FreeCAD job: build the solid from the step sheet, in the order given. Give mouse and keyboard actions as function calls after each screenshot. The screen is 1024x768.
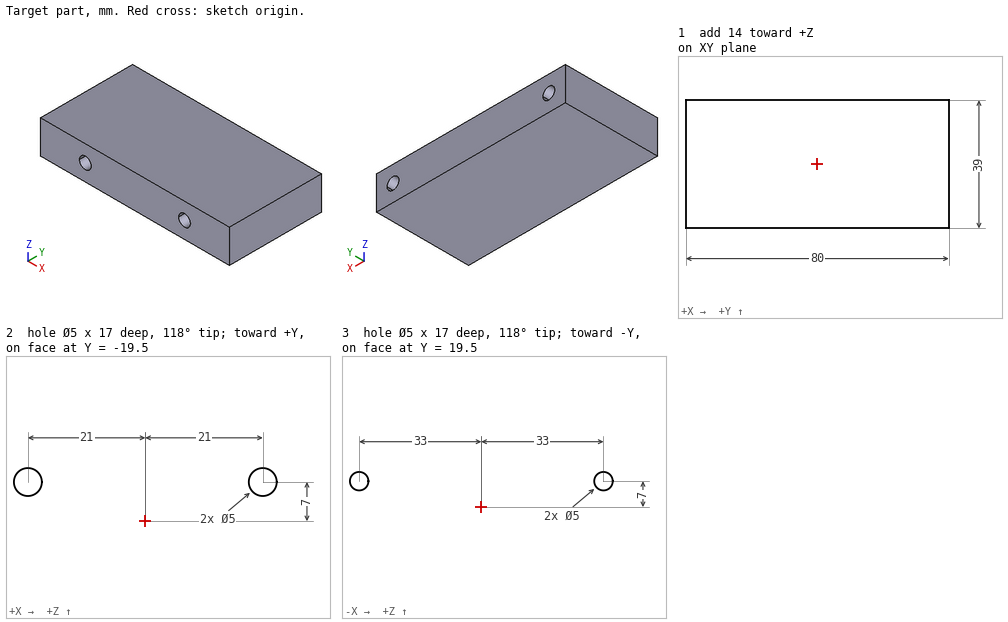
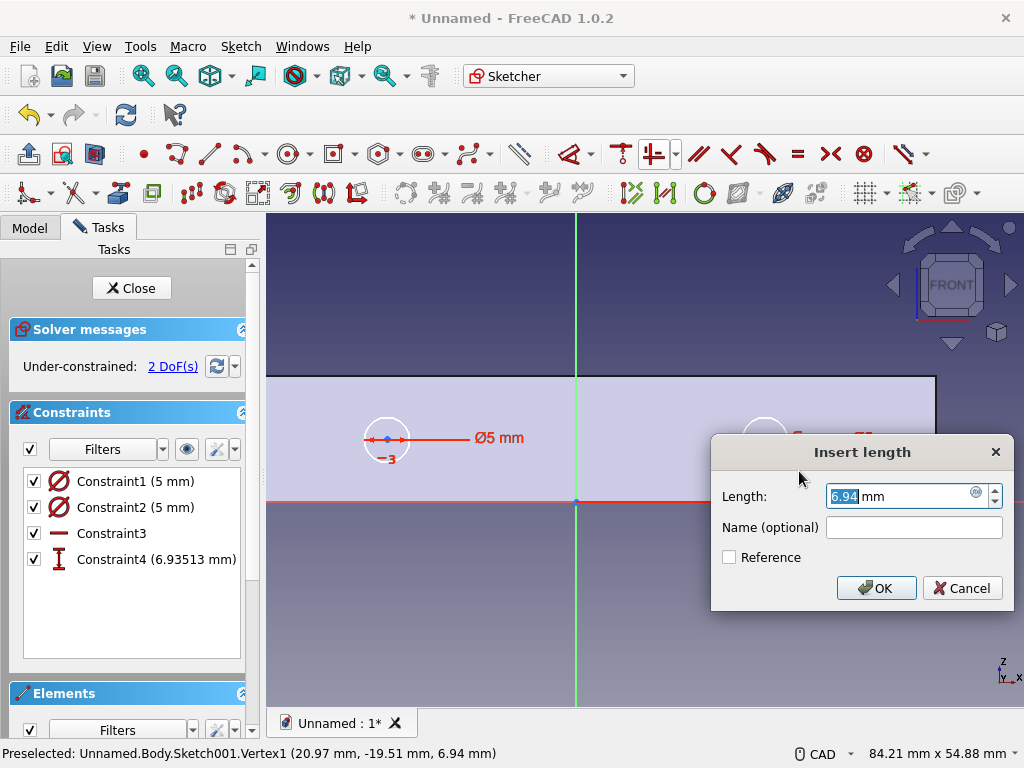
text(7)
key(Return)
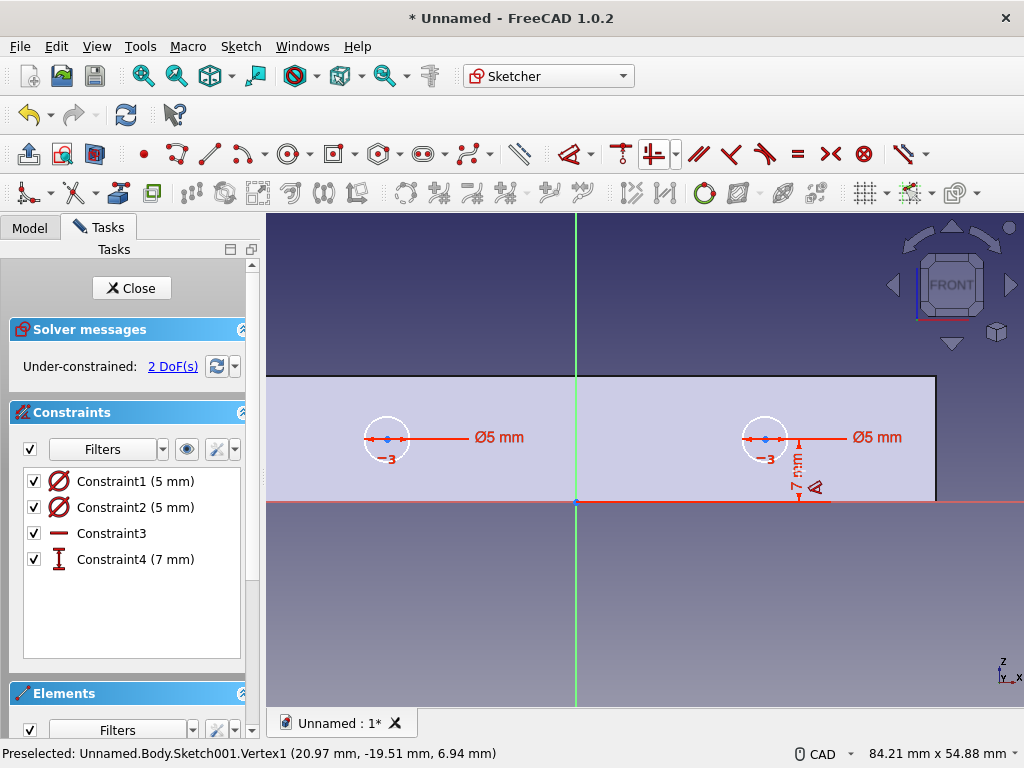
click(765, 439)
click(671, 536)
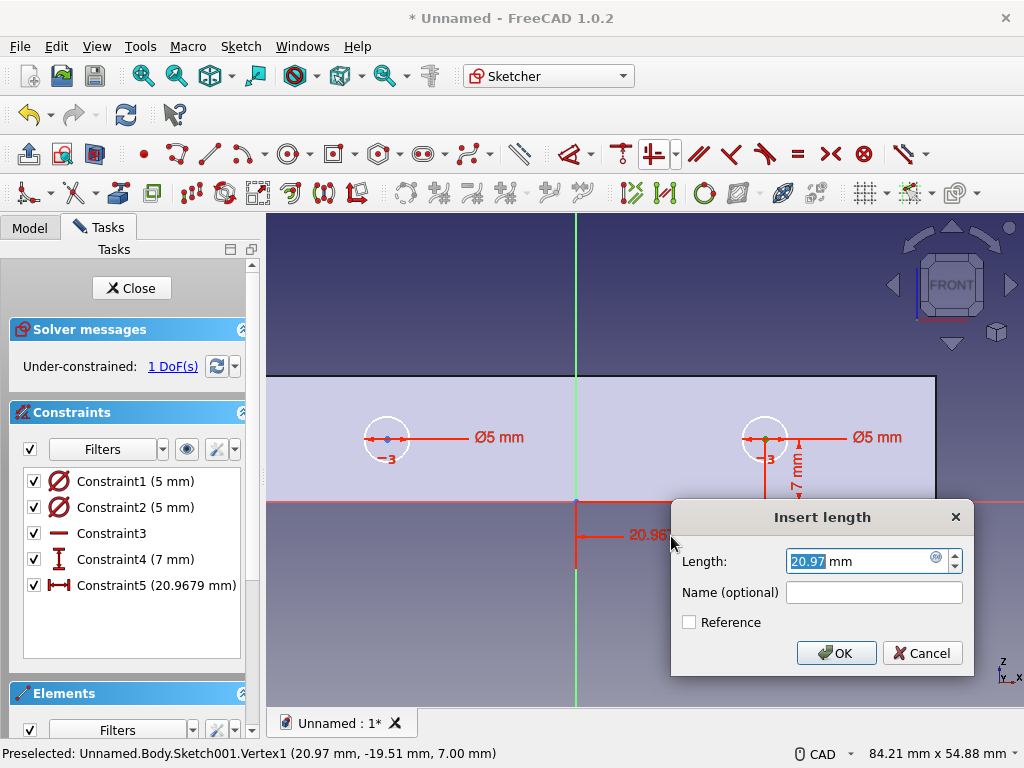
text(21)
key(Return)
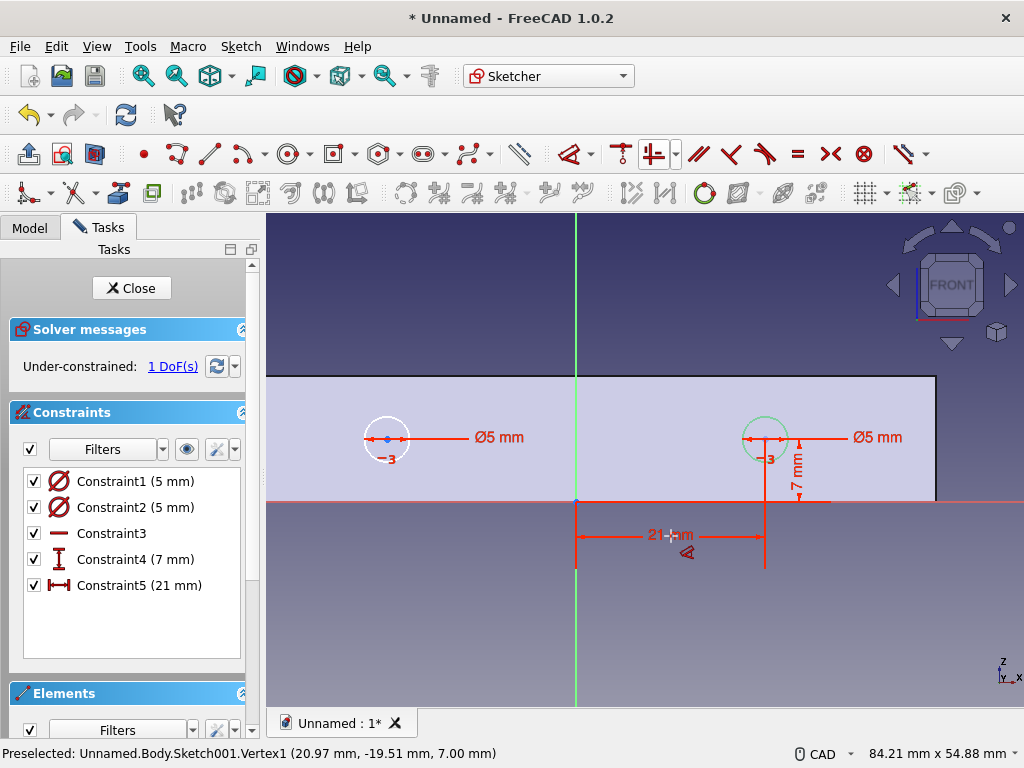
click(387, 439)
click(482, 536)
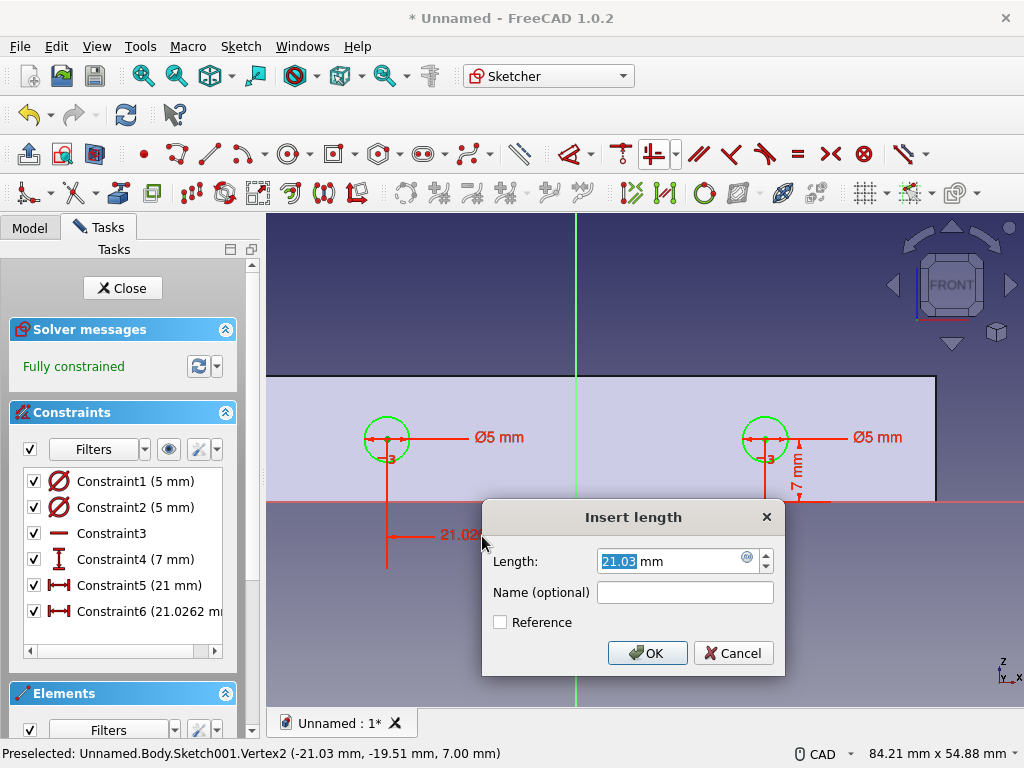
text(21)
key(Return)
key(Escape)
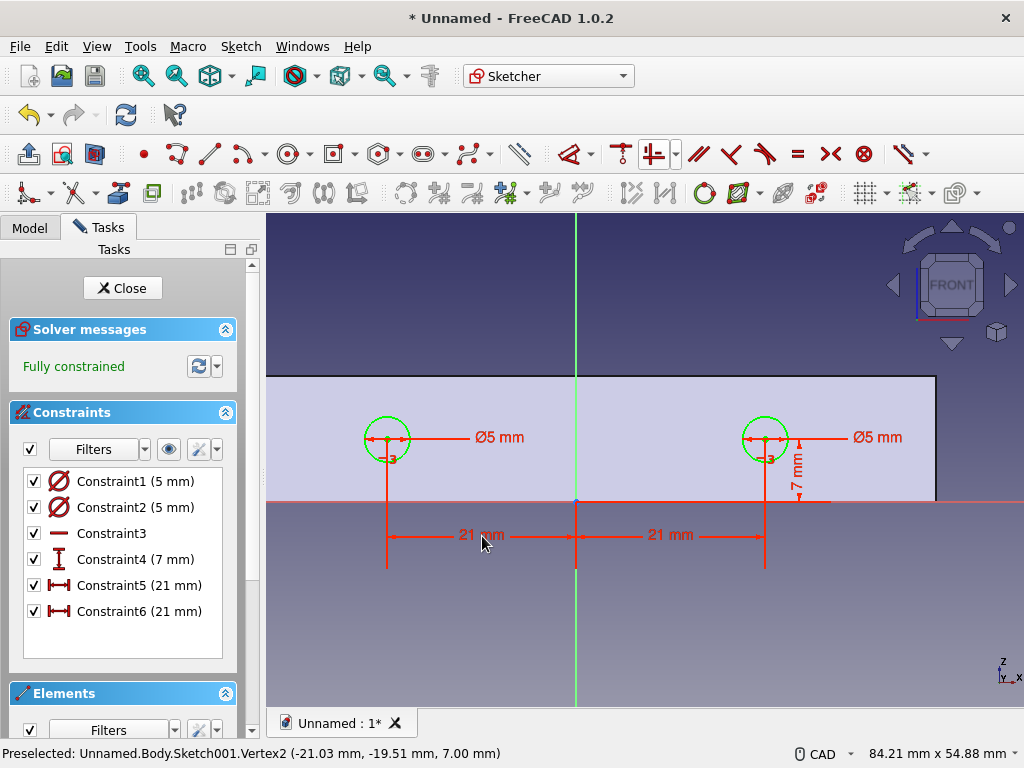
click(123, 288)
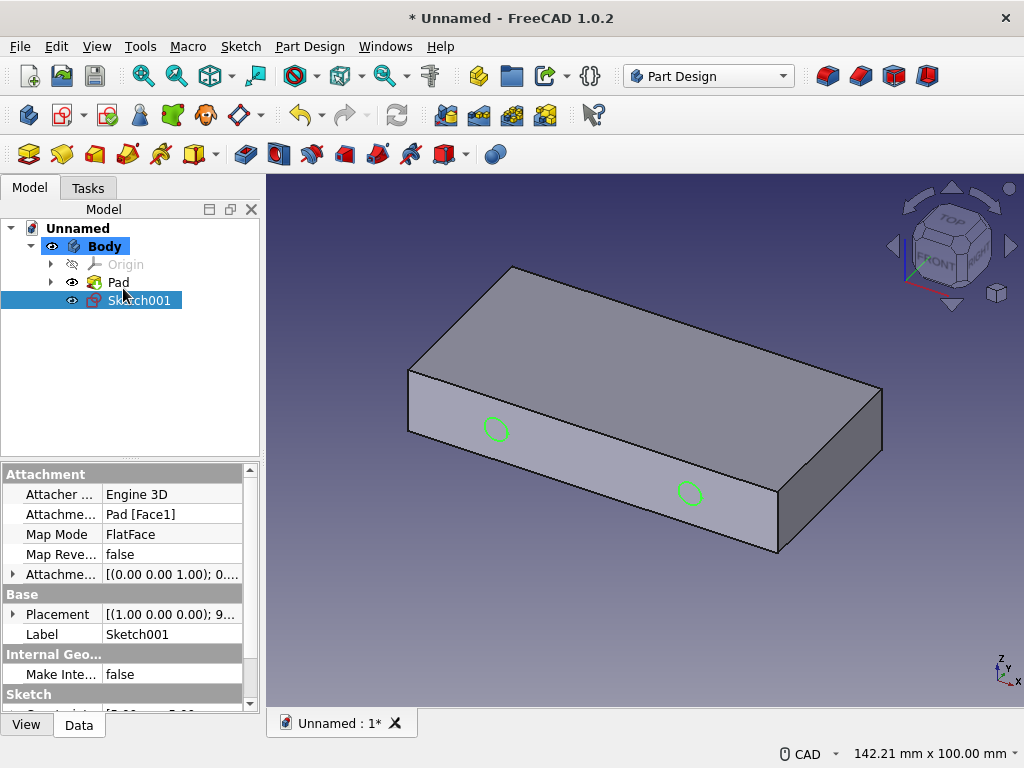
click(279, 154)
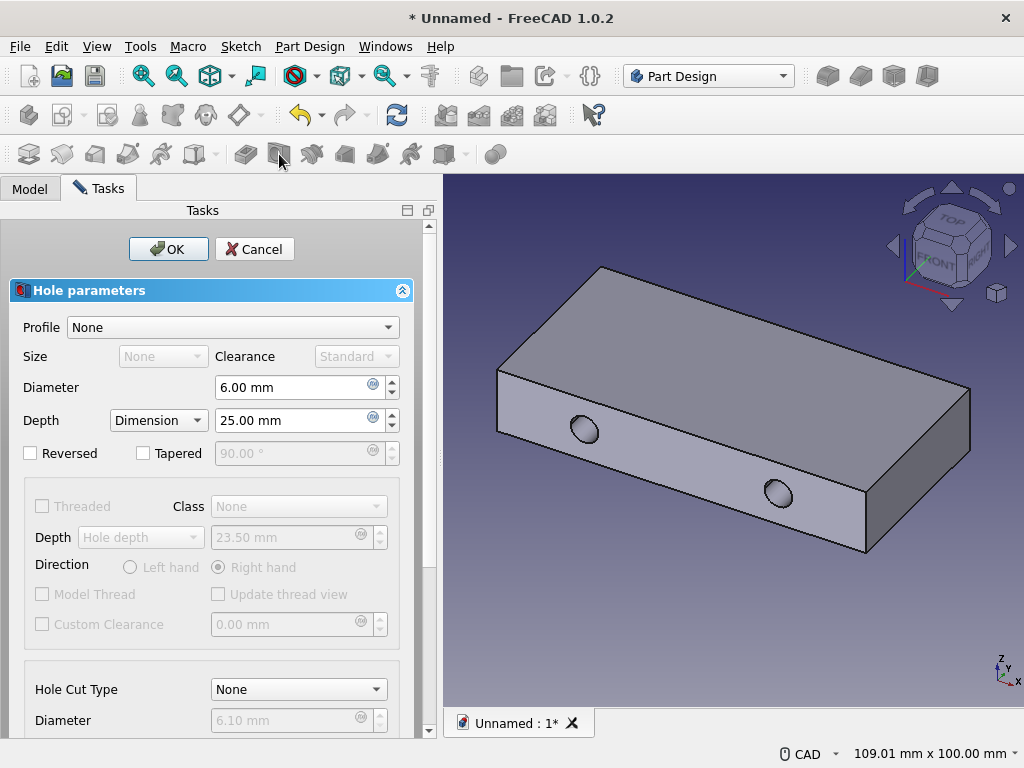
triple_click(300, 388)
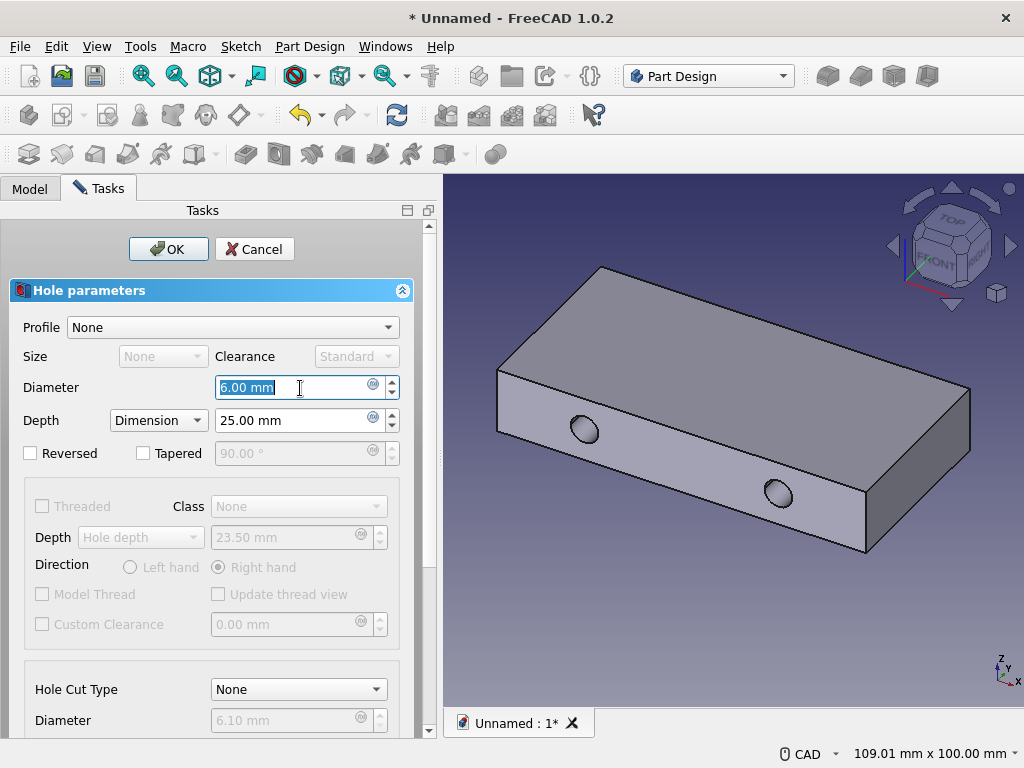
text(5)
key(Tab)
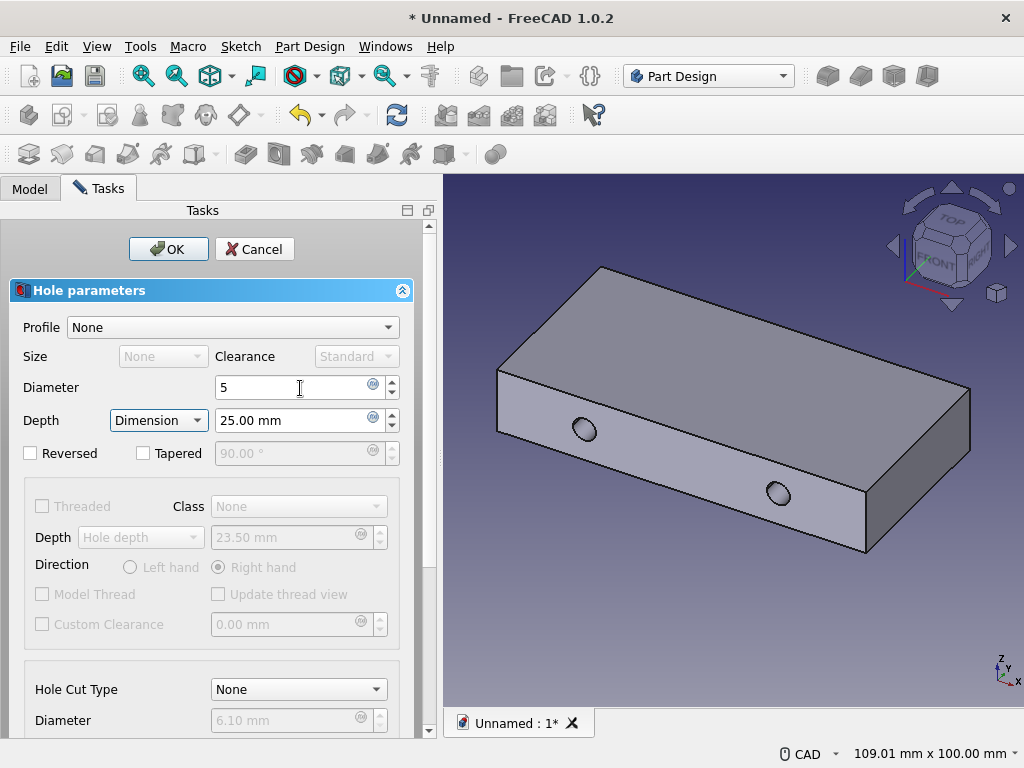
triple_click(300, 420)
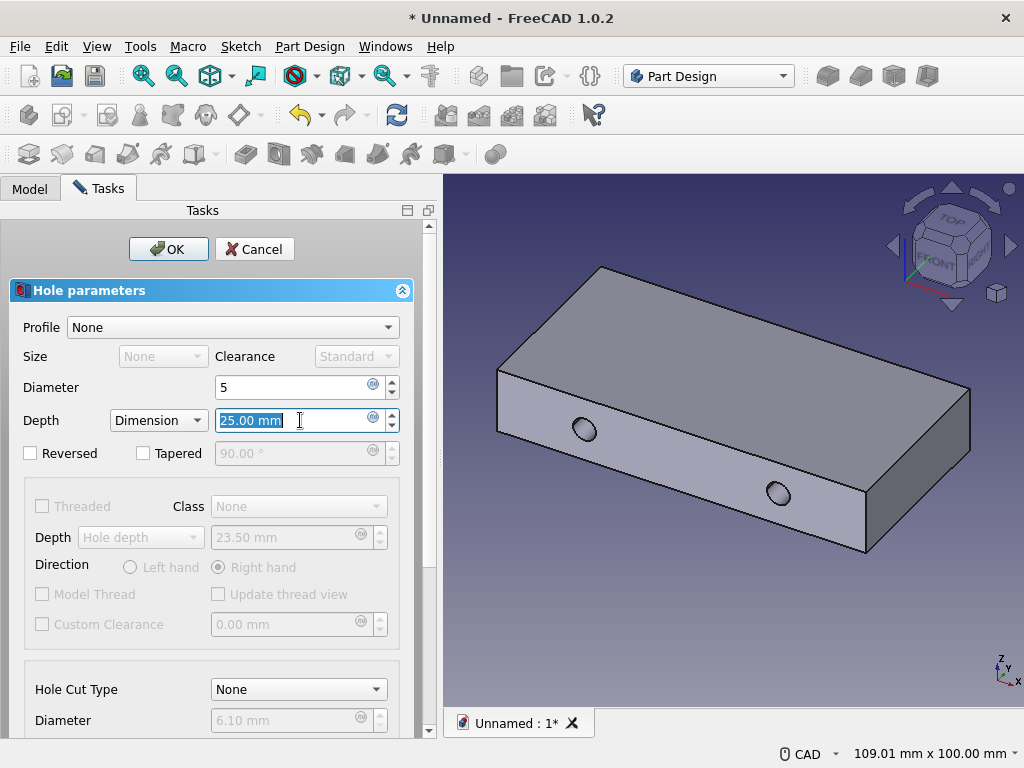
text(17)
key(Tab)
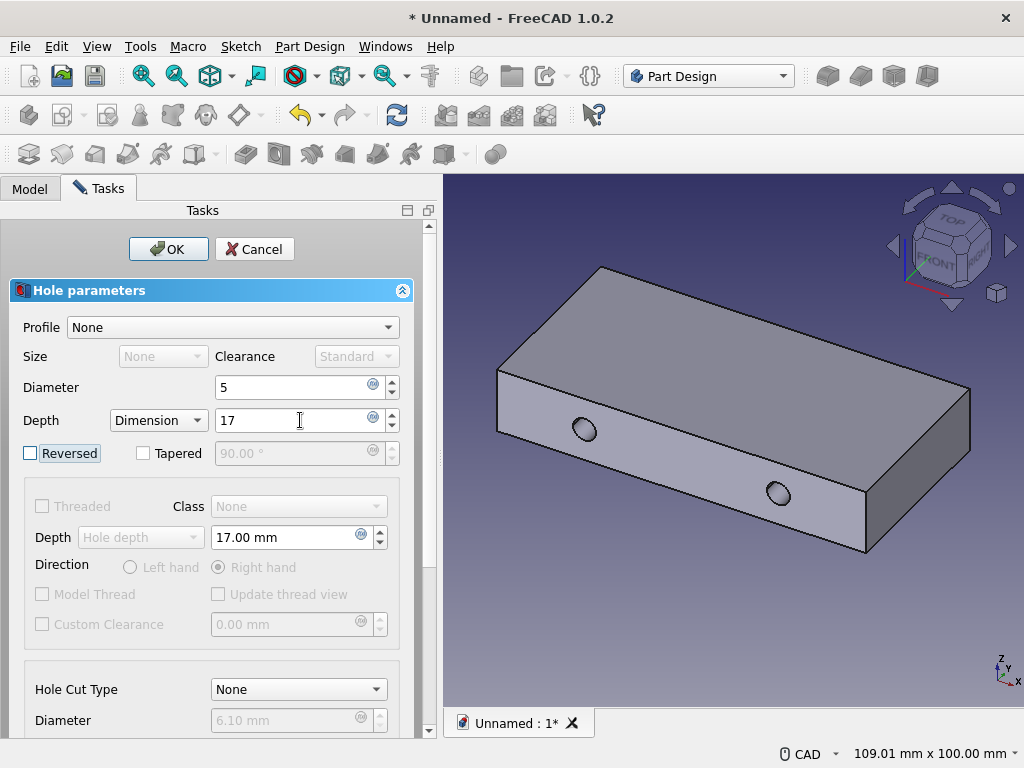
click(169, 249)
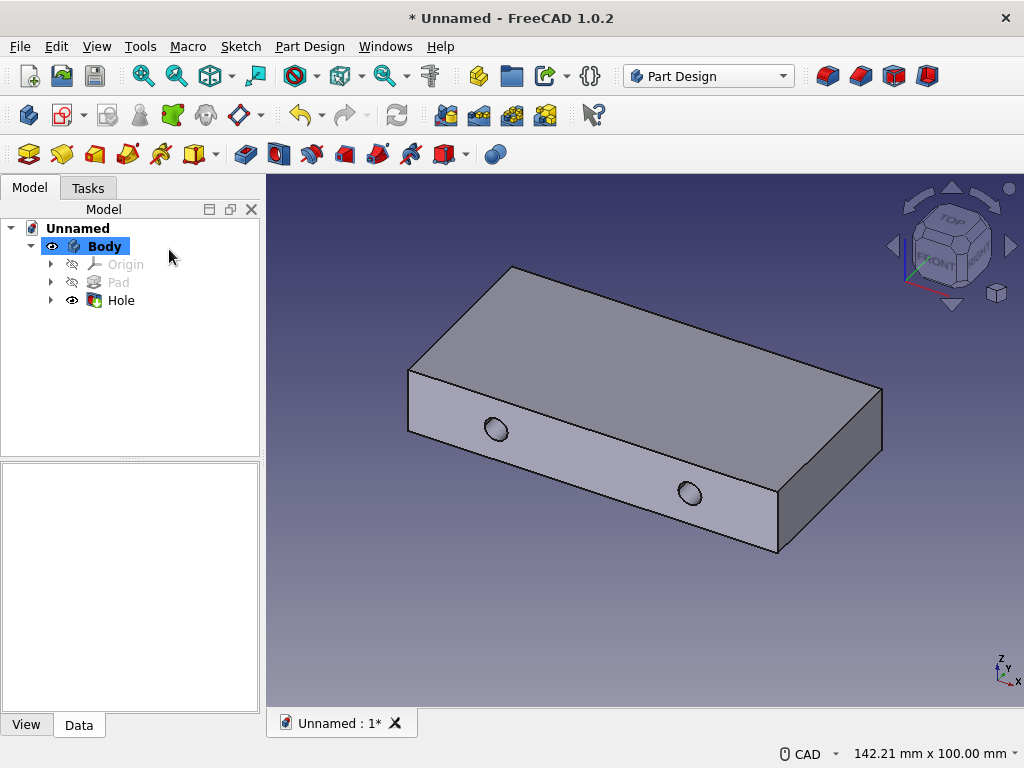
key(4)